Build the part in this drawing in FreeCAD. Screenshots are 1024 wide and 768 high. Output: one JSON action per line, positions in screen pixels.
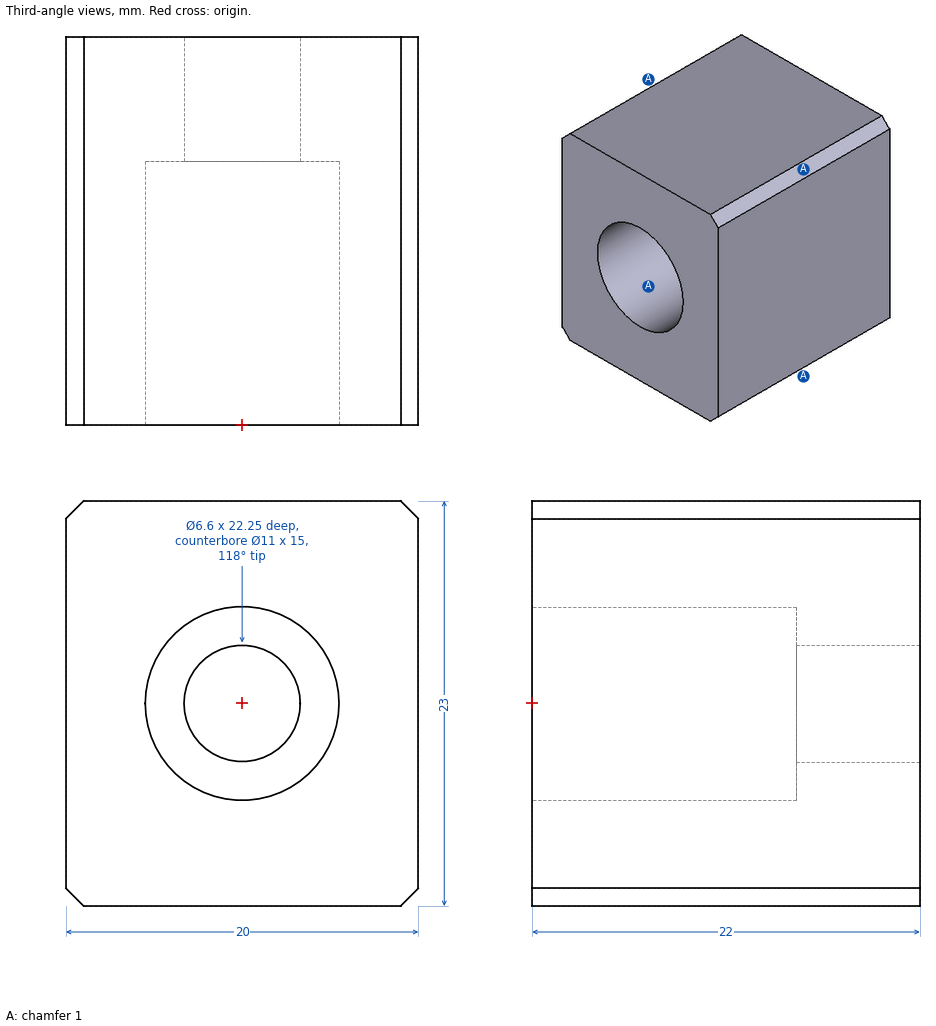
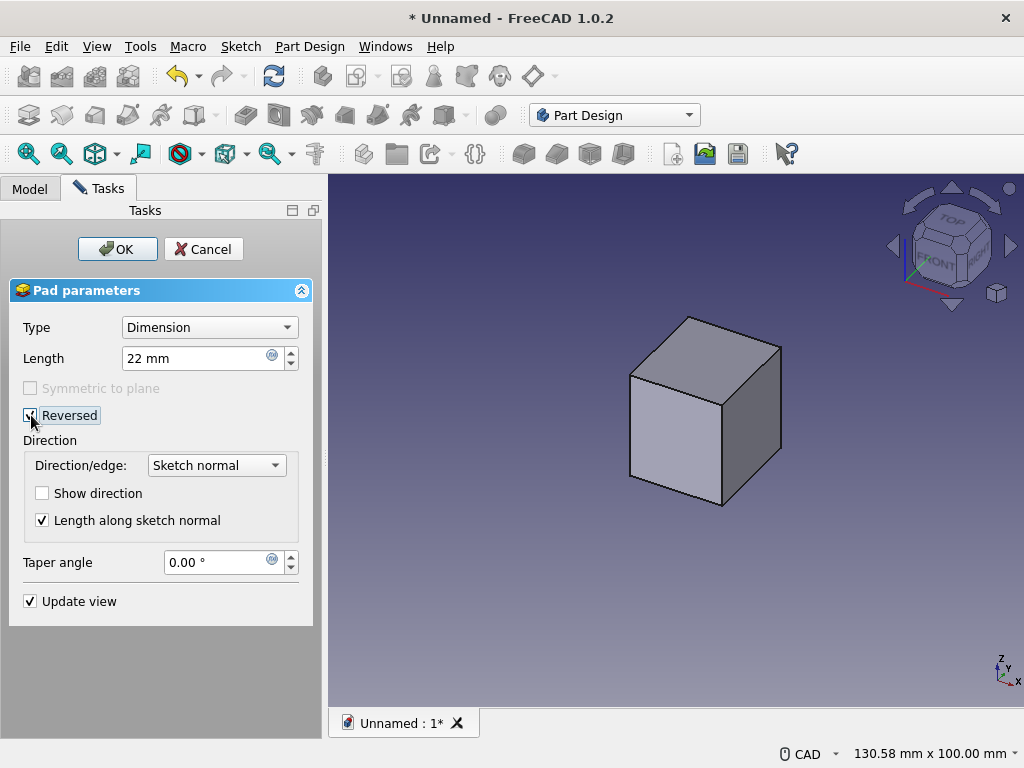
{"action": "left_click", "coordinate": [118, 249]}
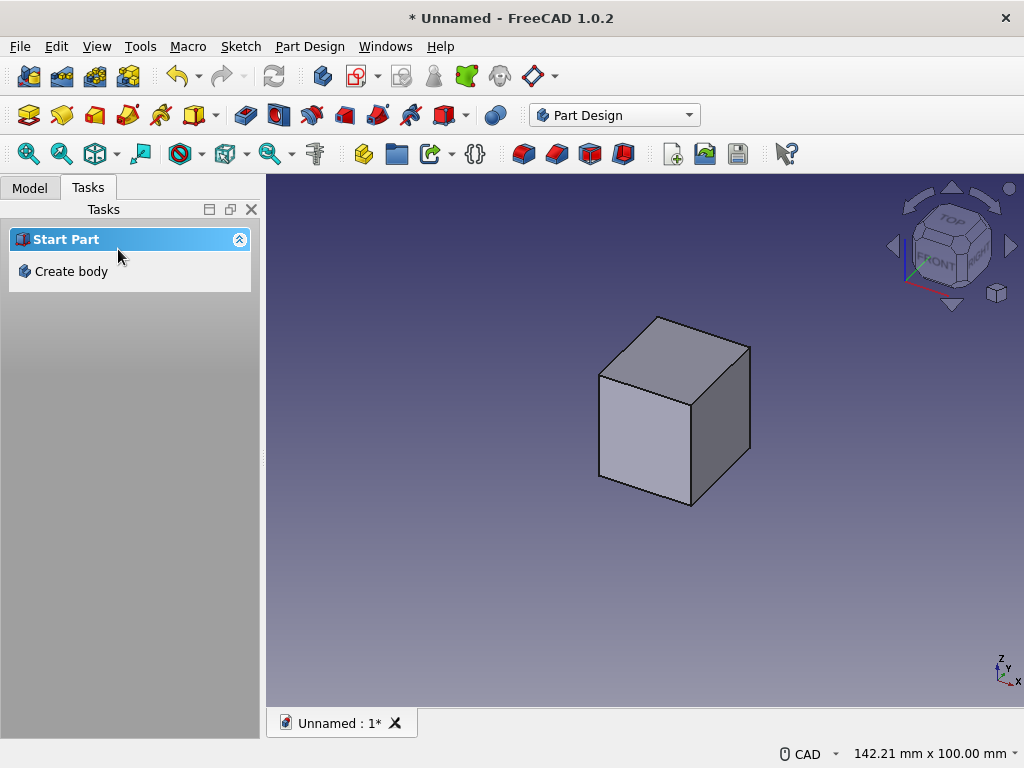
{"action": "key", "text": "v f"}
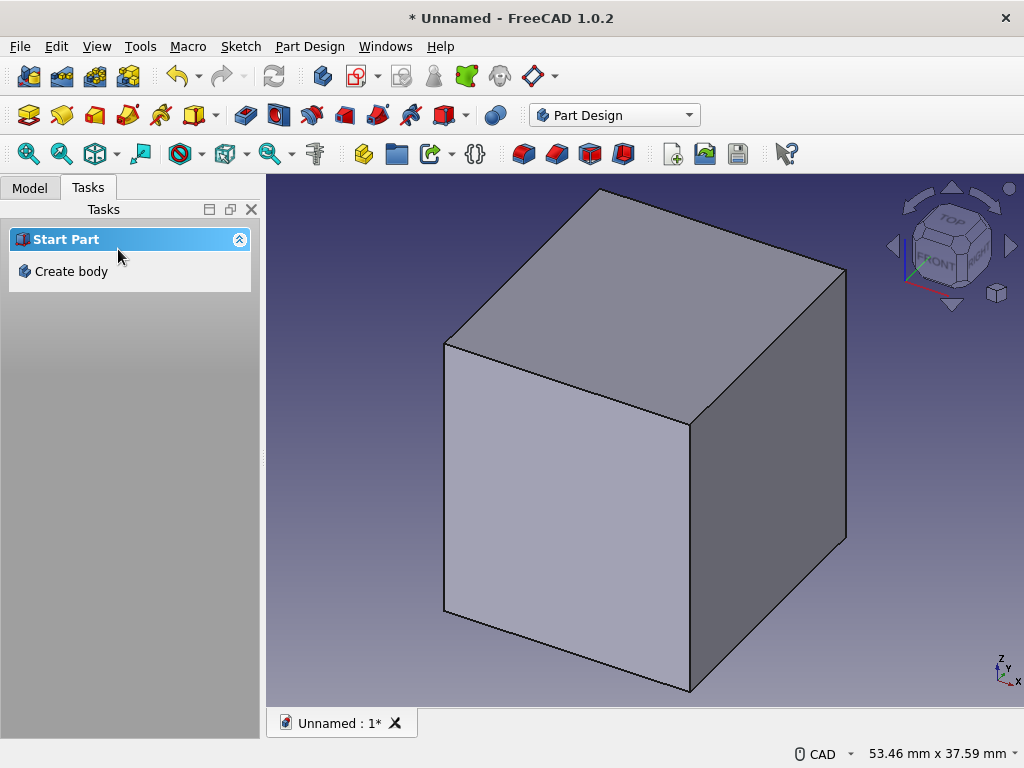
{"action": "left_click", "coordinate": [567, 517]}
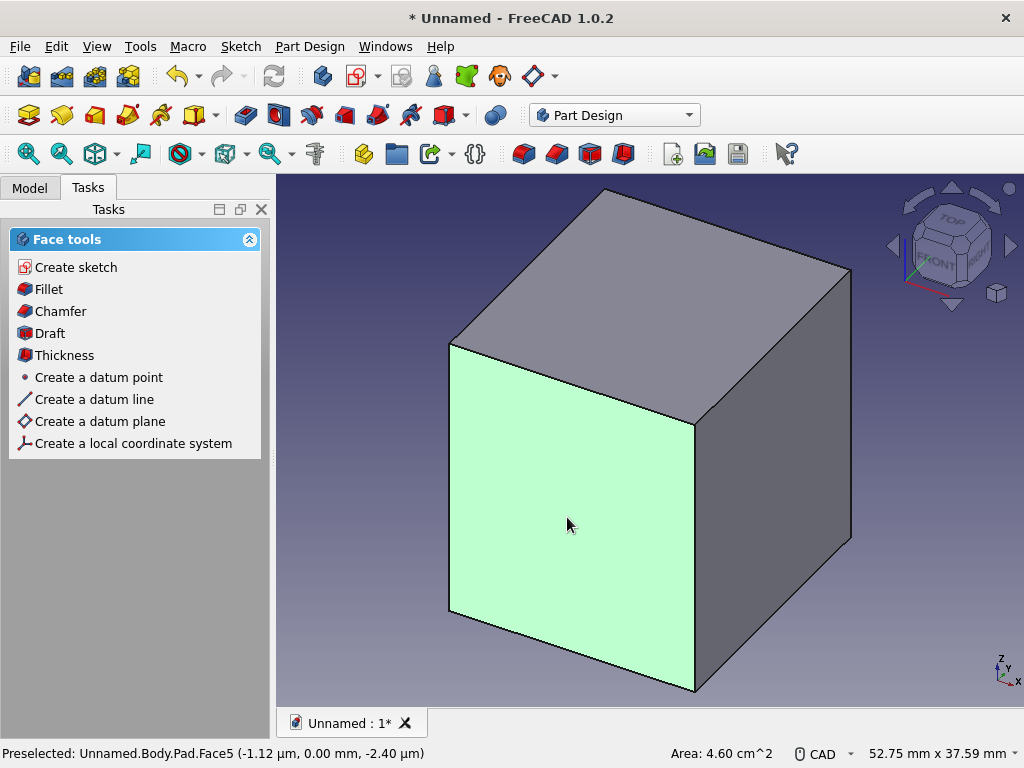
{"action": "left_click", "coordinate": [356, 76]}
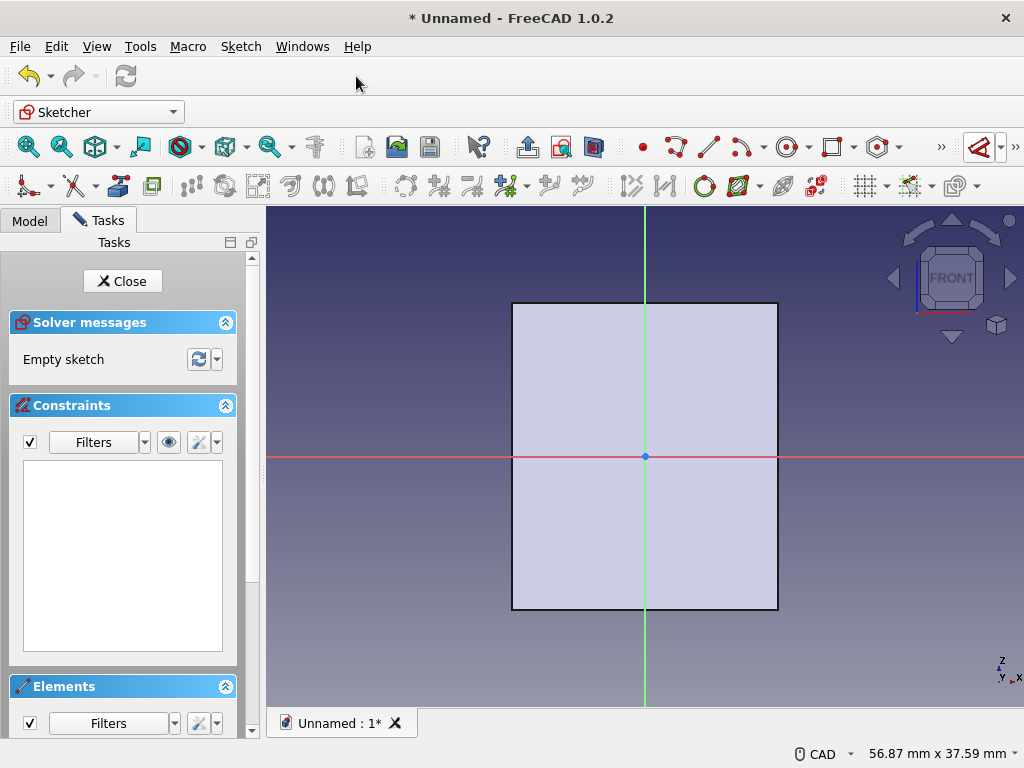
{"action": "scroll", "coordinate": [675, 457], "scroll_direction": "up", "scroll_amount": 6}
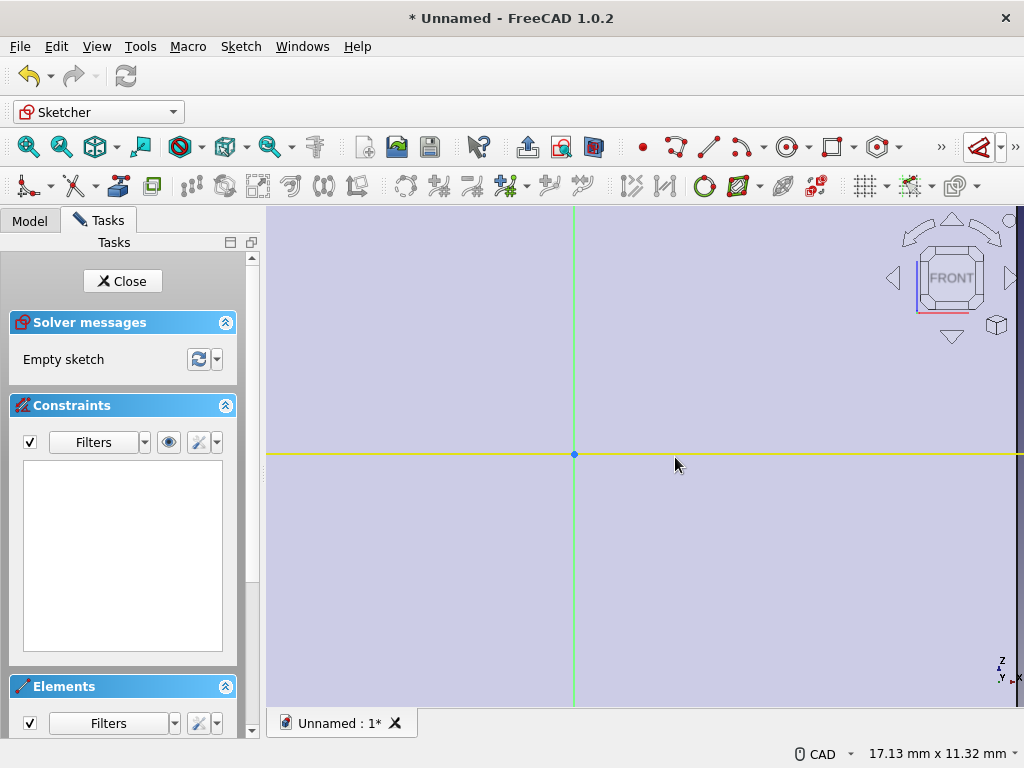
{"action": "key", "text": "g c"}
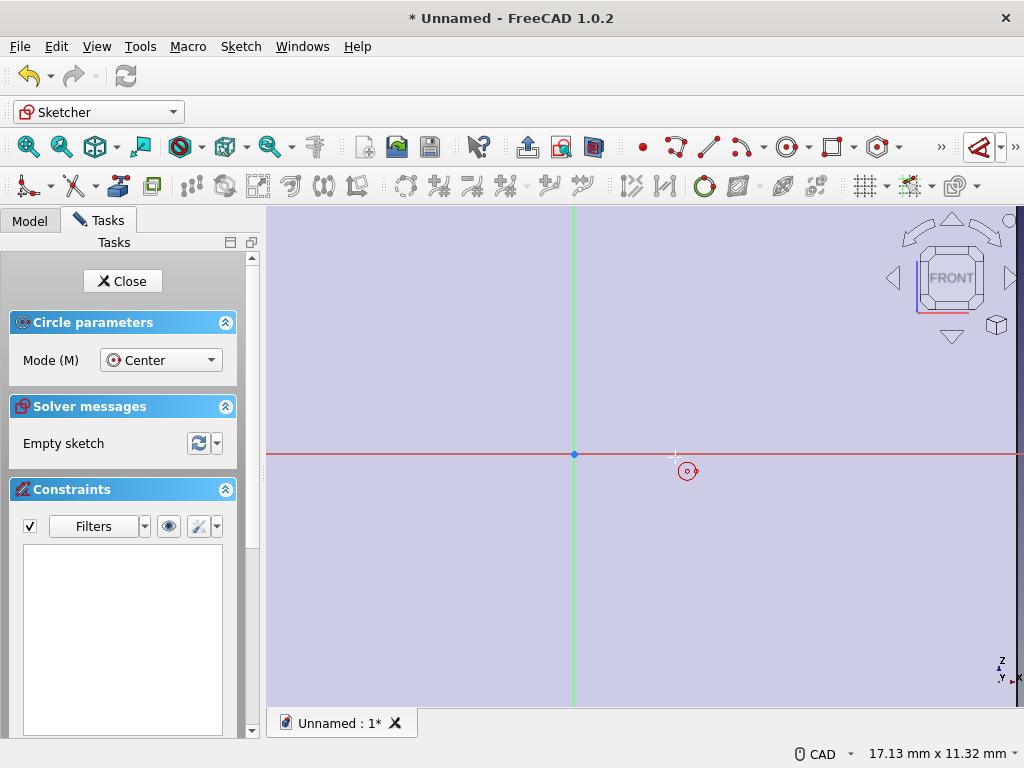
{"action": "left_click", "coordinate": [574, 454]}
{"action": "mouse_move", "coordinate": [677, 351]}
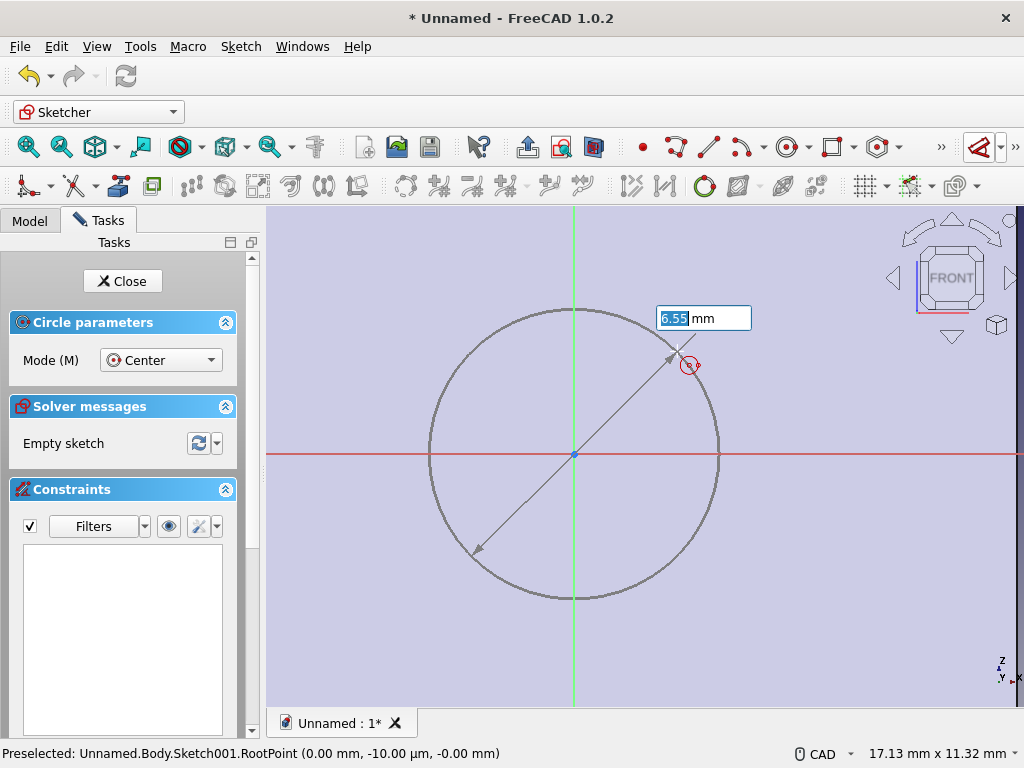
{"action": "type", "text": "6.6"}
{"action": "key", "text": "Return"}
{"action": "key", "text": "Escape"}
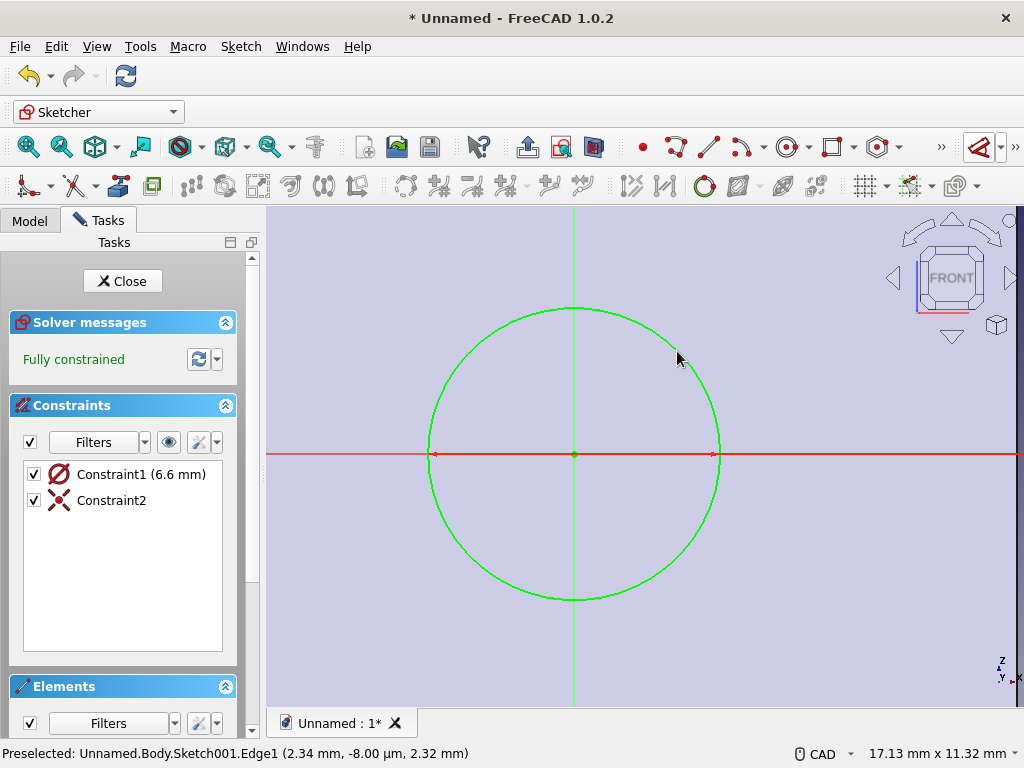
{"action": "left_click", "coordinate": [123, 281]}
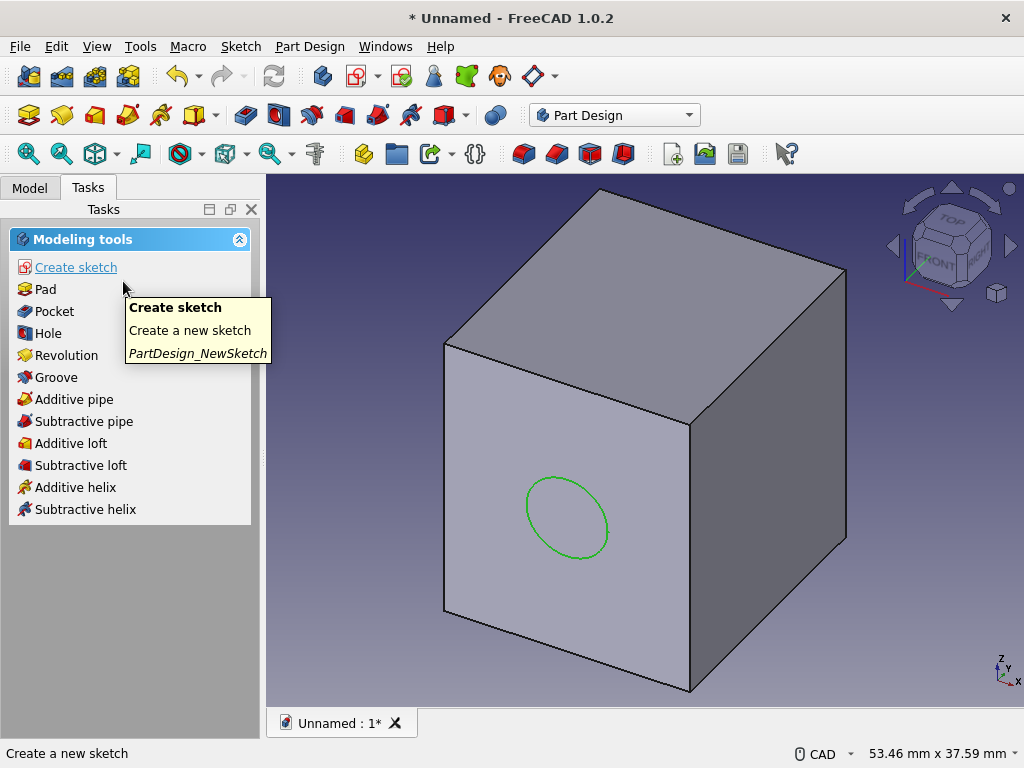
{"action": "left_click", "coordinate": [279, 116]}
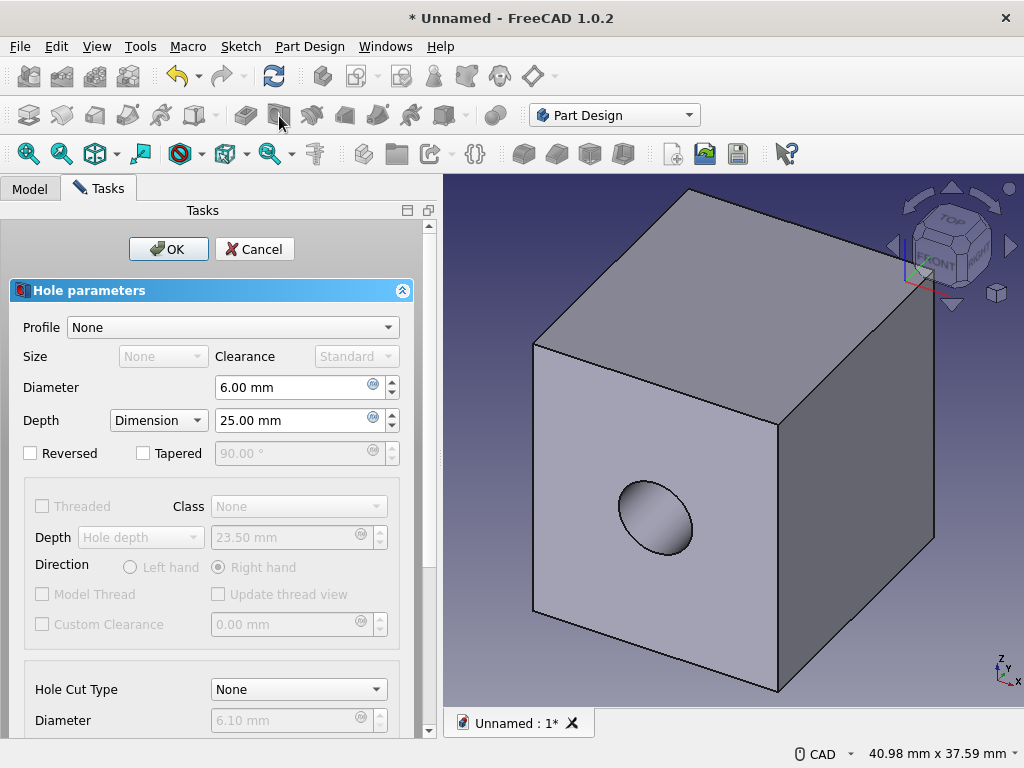
{"action": "triple_click", "coordinate": [300, 388]}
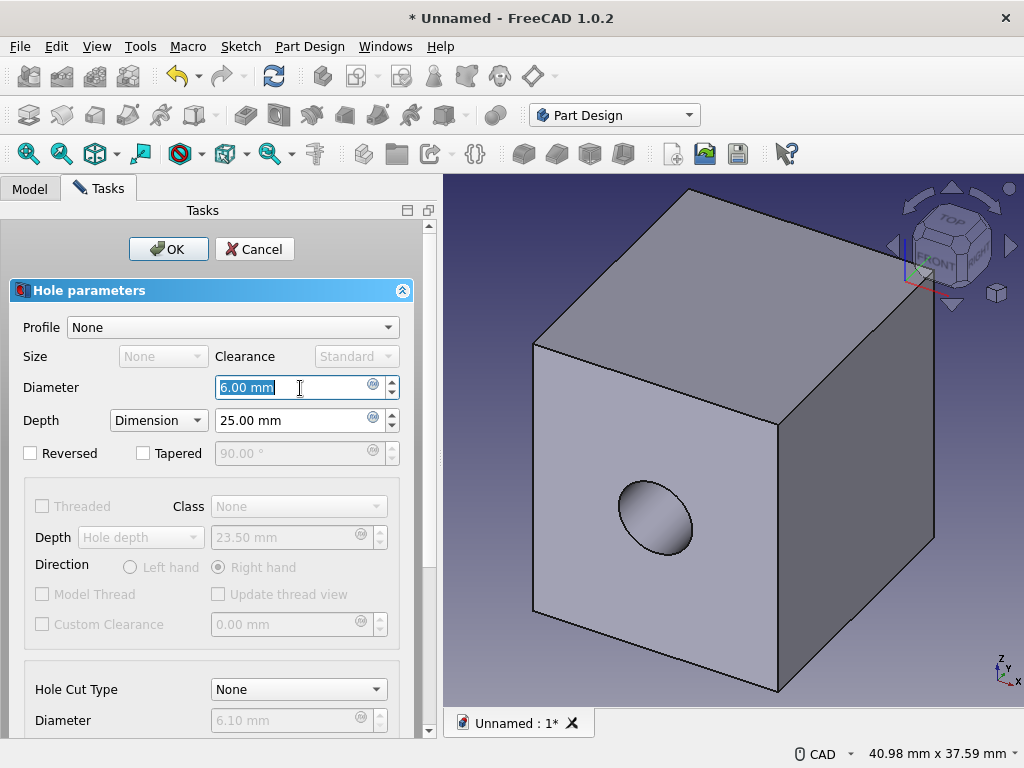
{"action": "type", "text": "6.6"}
{"action": "key", "text": "Tab"}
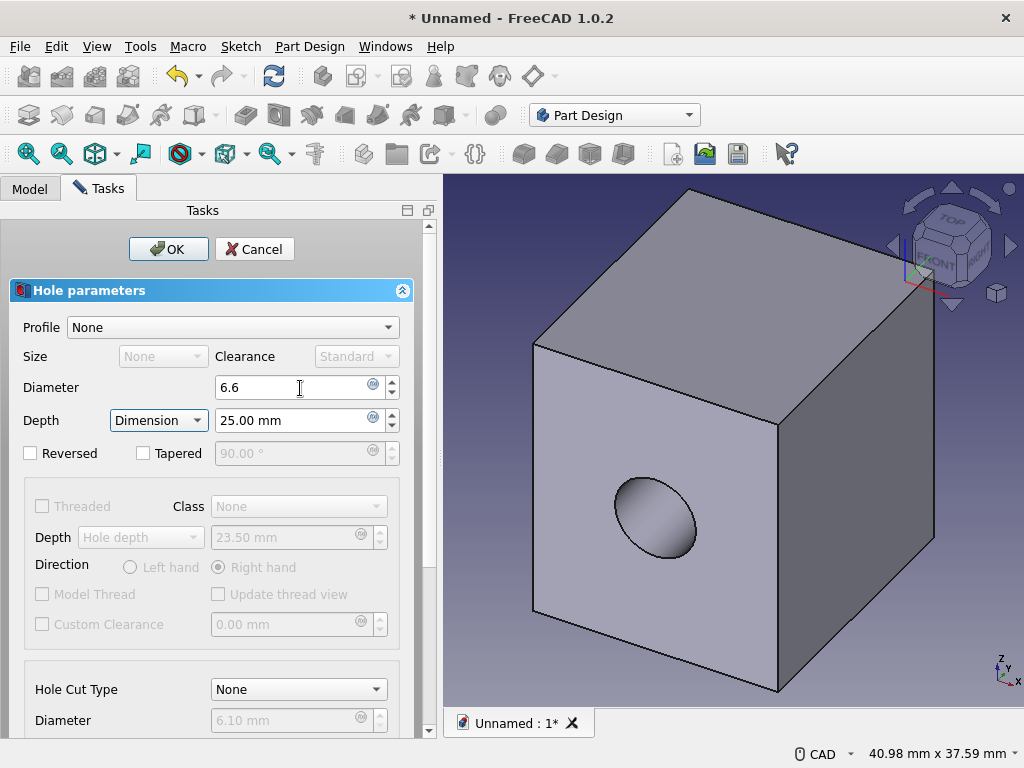
{"action": "triple_click", "coordinate": [300, 420]}